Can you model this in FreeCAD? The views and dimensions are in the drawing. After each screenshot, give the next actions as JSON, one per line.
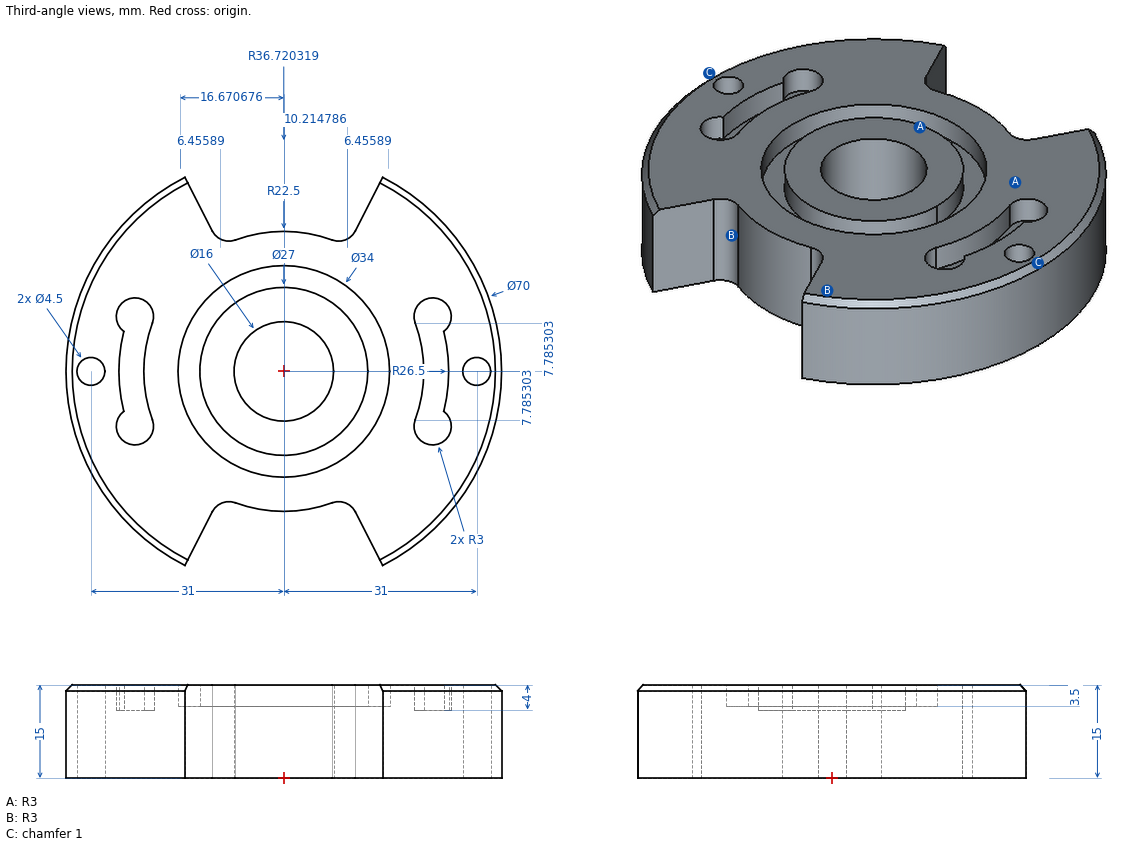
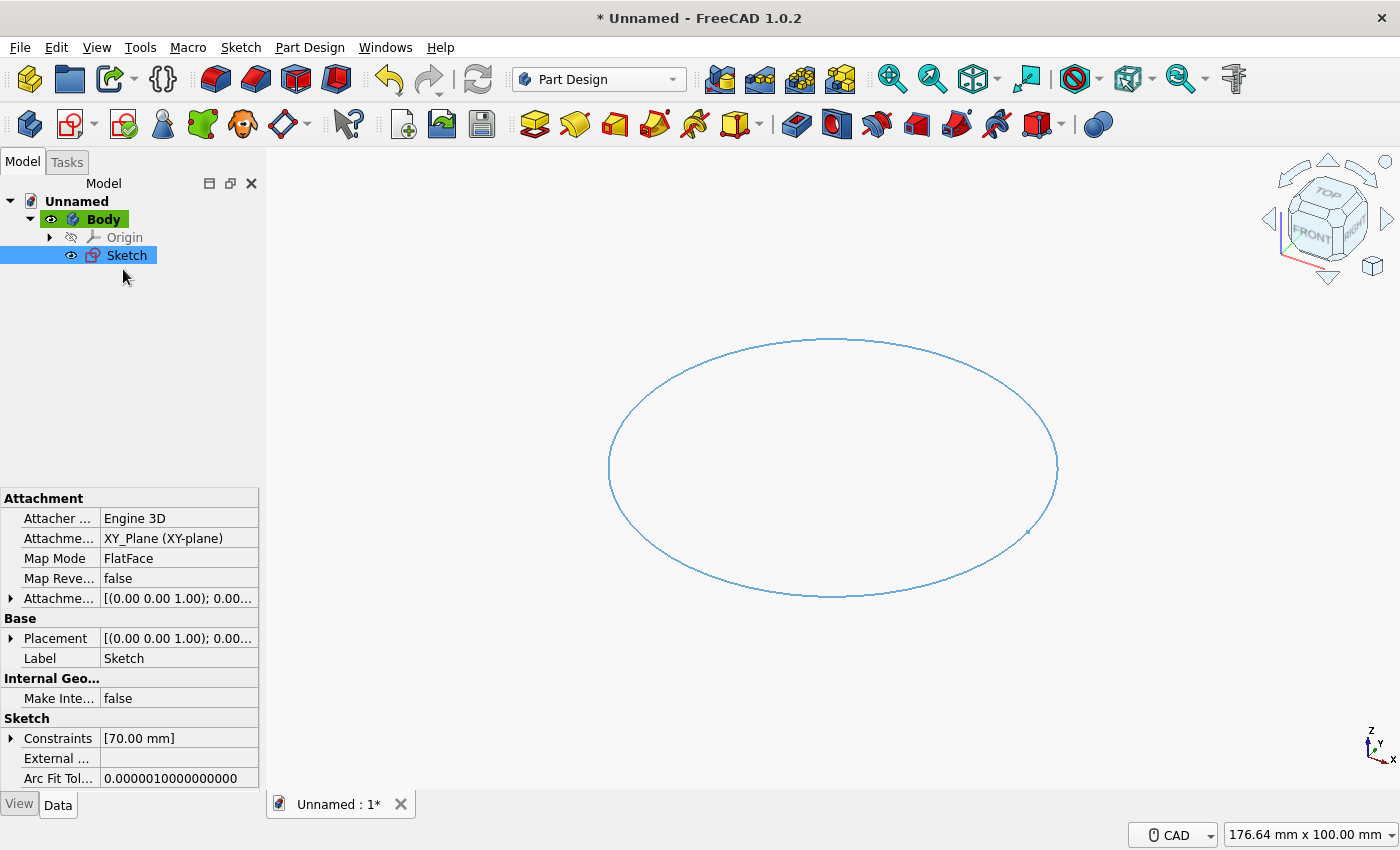
{"action": "left_click", "coordinate": [536, 124]}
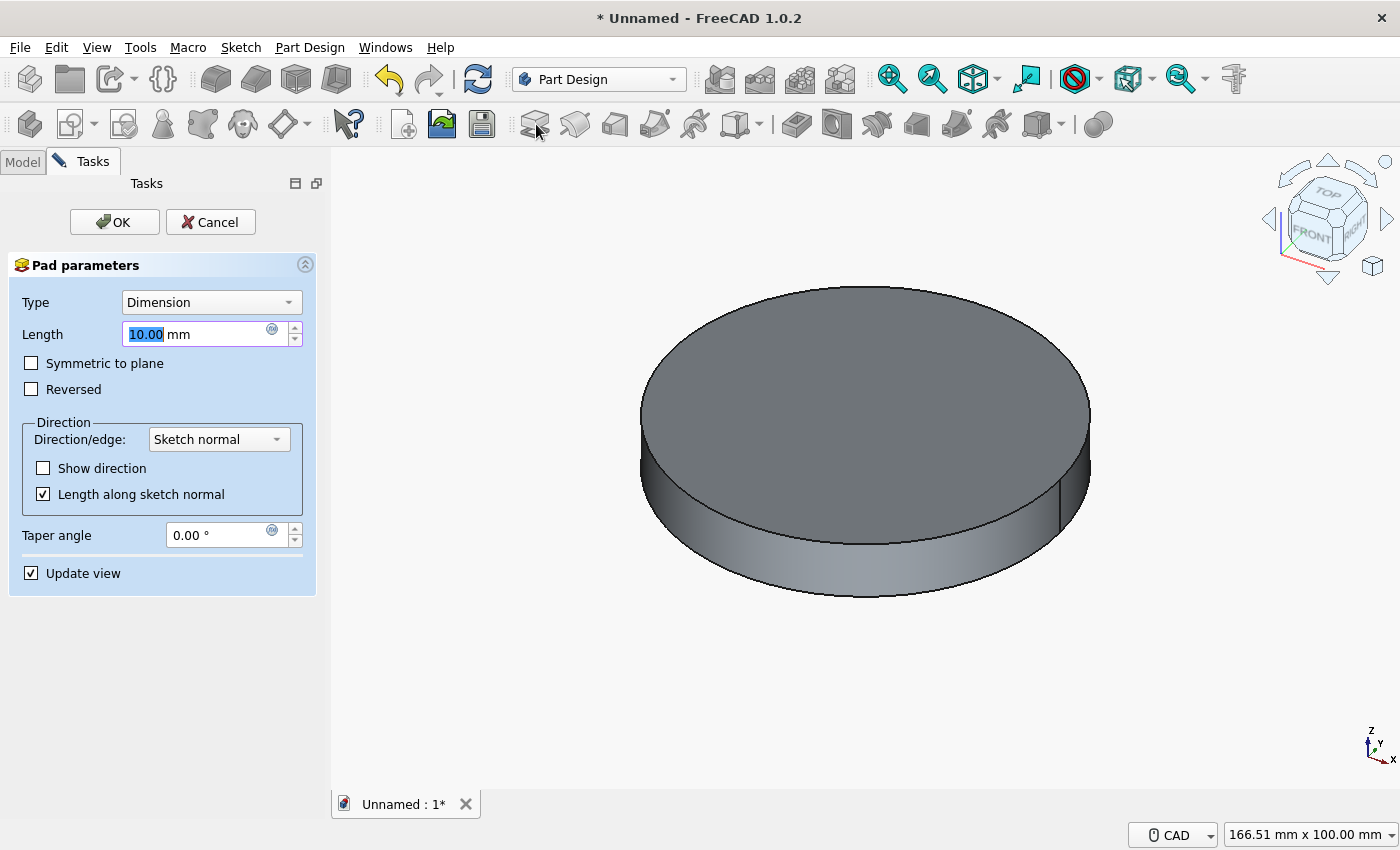
{"action": "type", "text": "15"}
{"action": "key", "text": "Tab"}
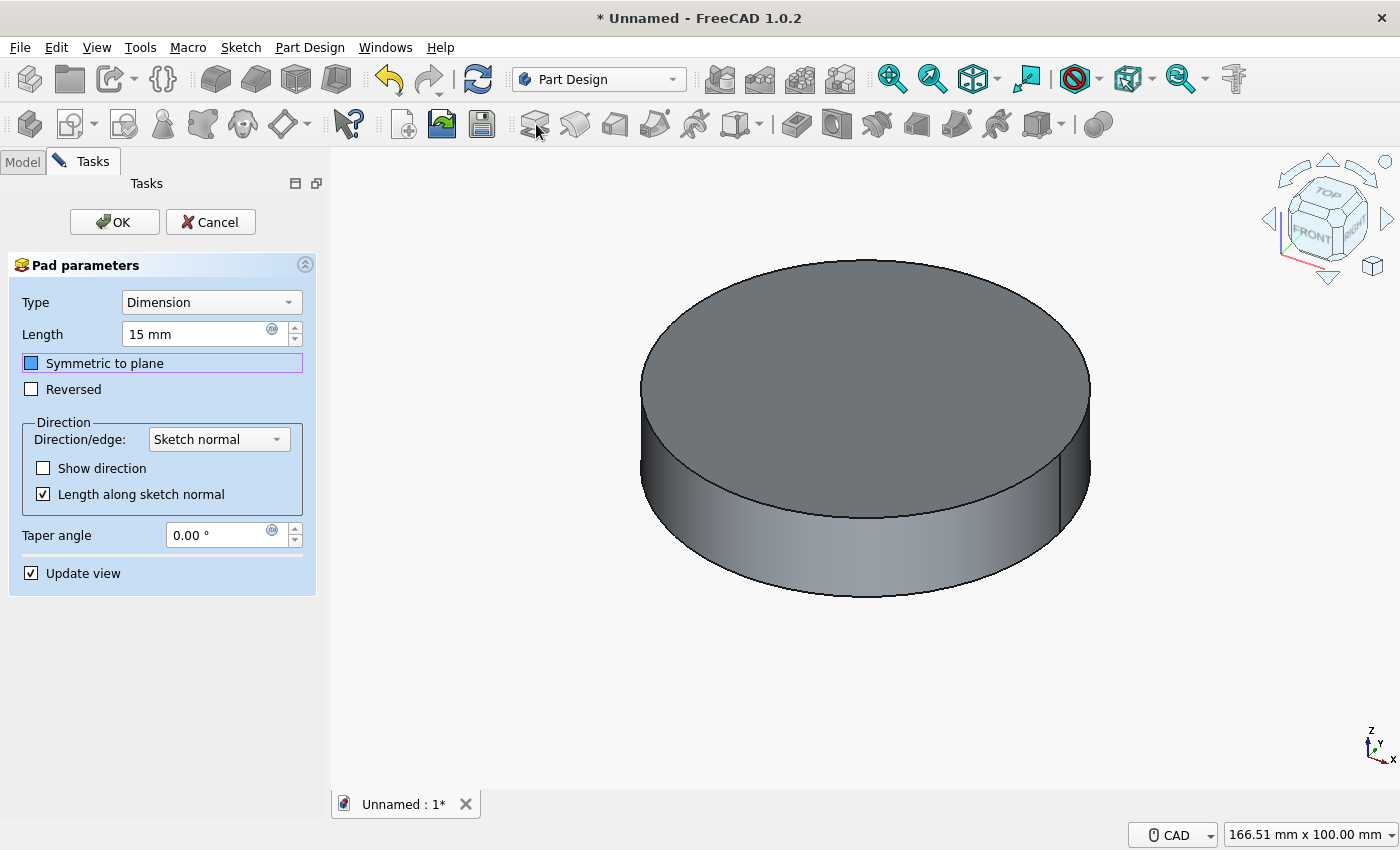
{"action": "left_click", "coordinate": [115, 222]}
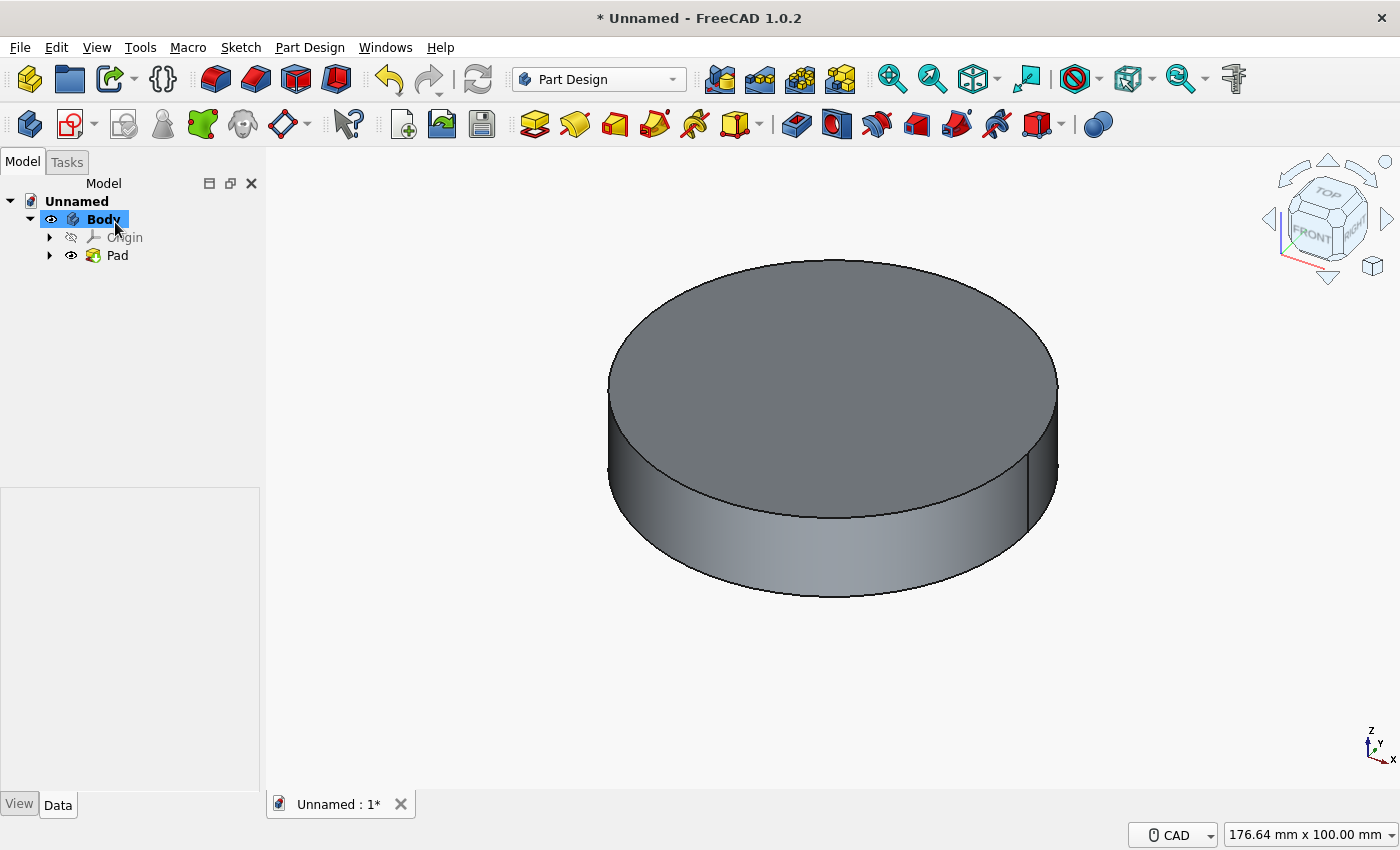
{"action": "left_click", "coordinate": [833, 388]}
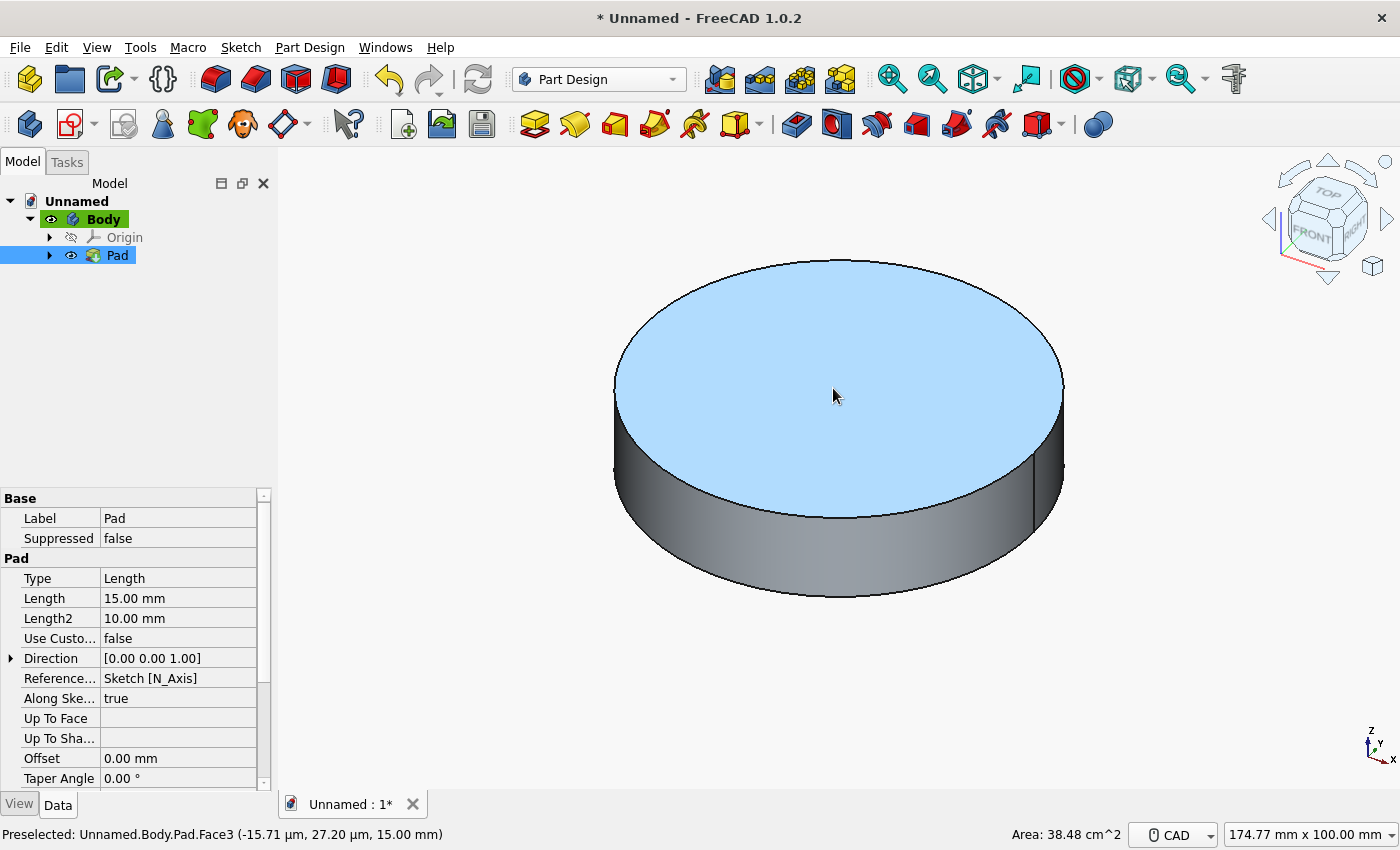
{"action": "left_click", "coordinate": [70, 124]}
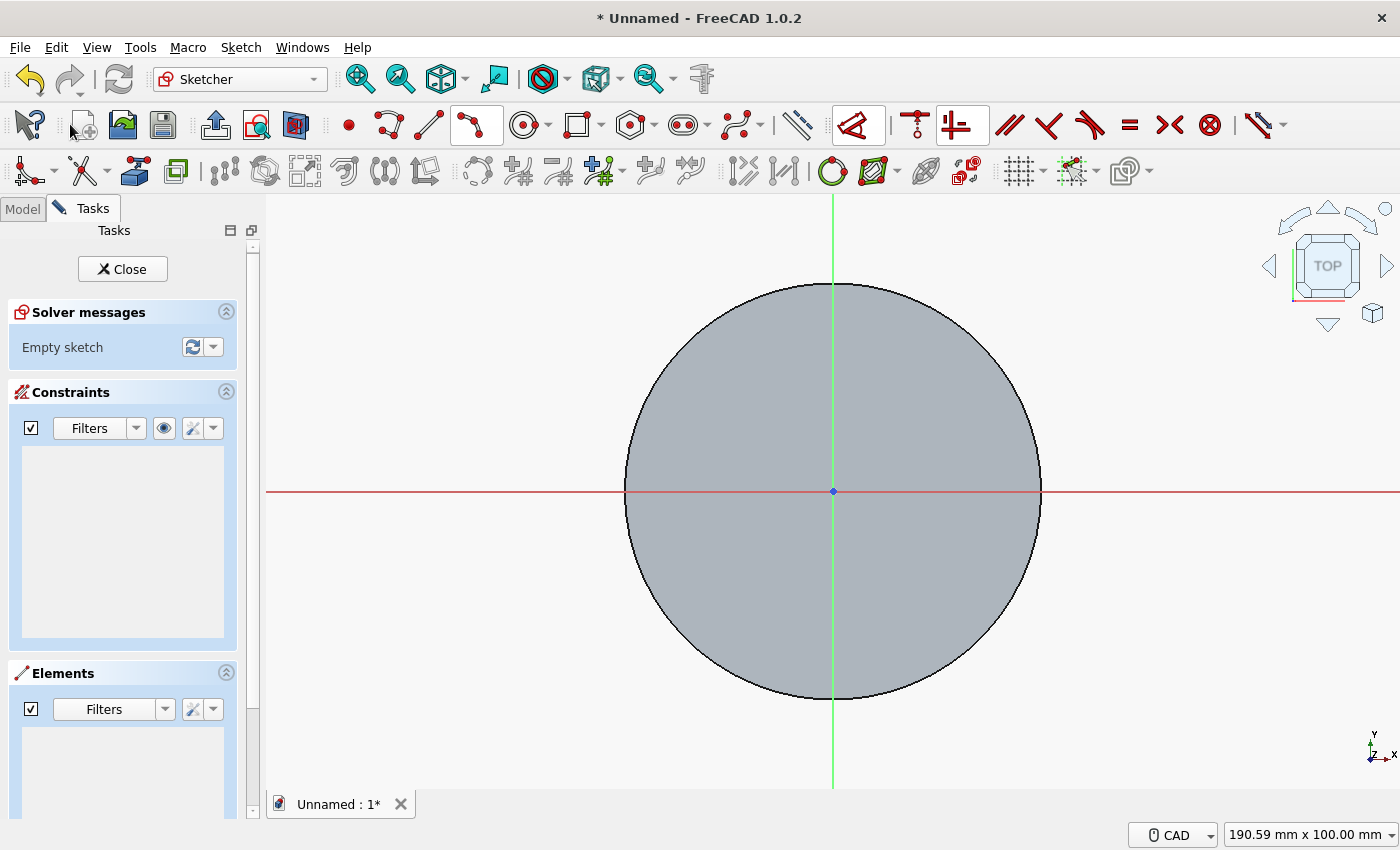
{"action": "scroll", "coordinate": [916, 249], "scroll_direction": "up", "scroll_amount": 3}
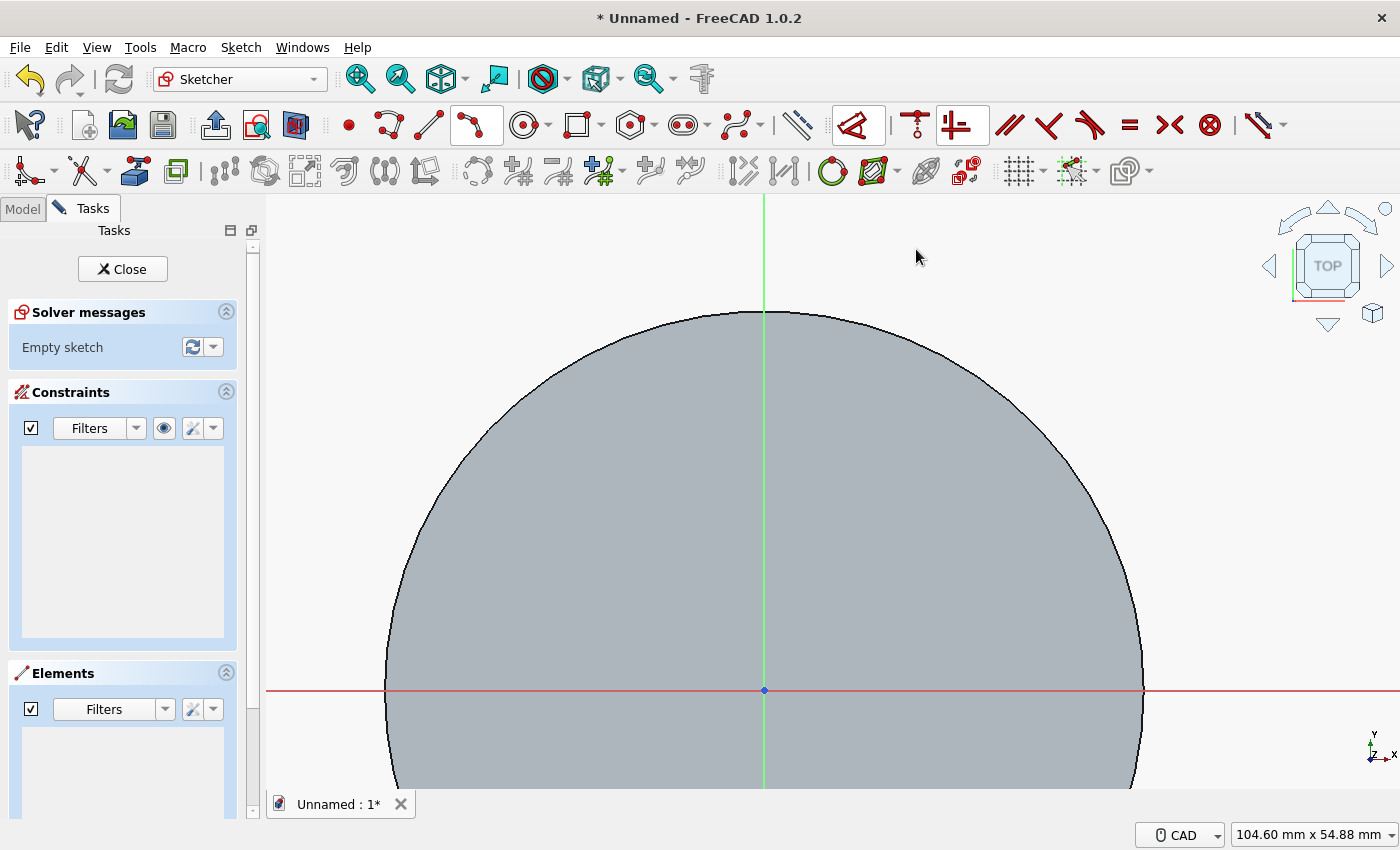
{"action": "key", "text": "g l"}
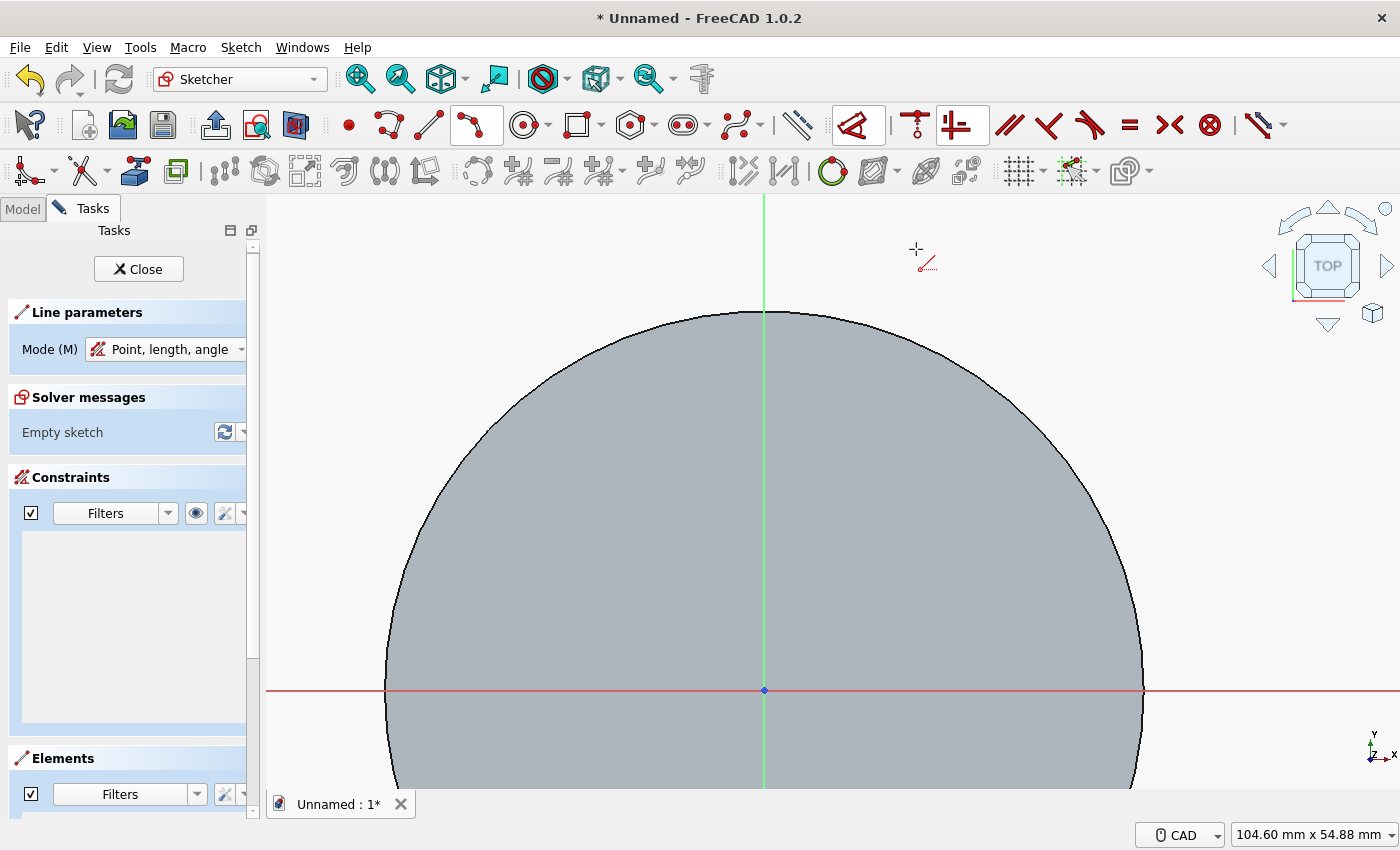
{"action": "left_click", "coordinate": [584, 336]}
{"action": "left_click", "coordinate": [654, 473]}